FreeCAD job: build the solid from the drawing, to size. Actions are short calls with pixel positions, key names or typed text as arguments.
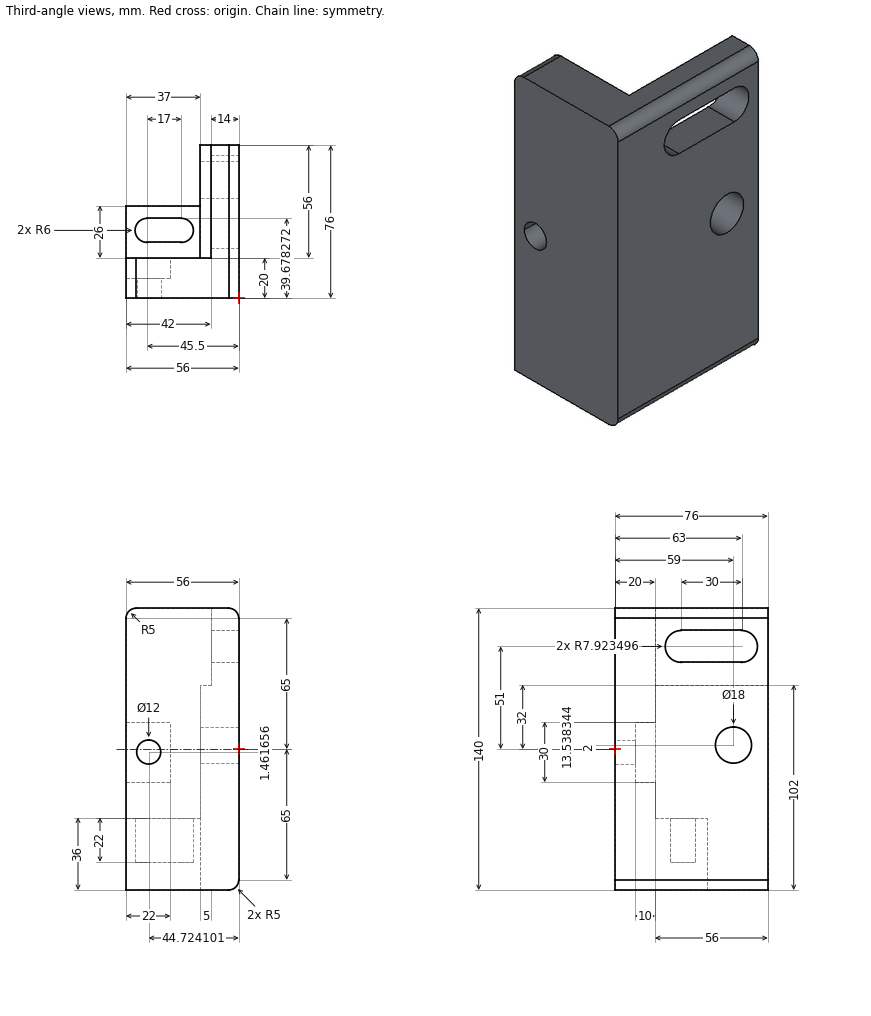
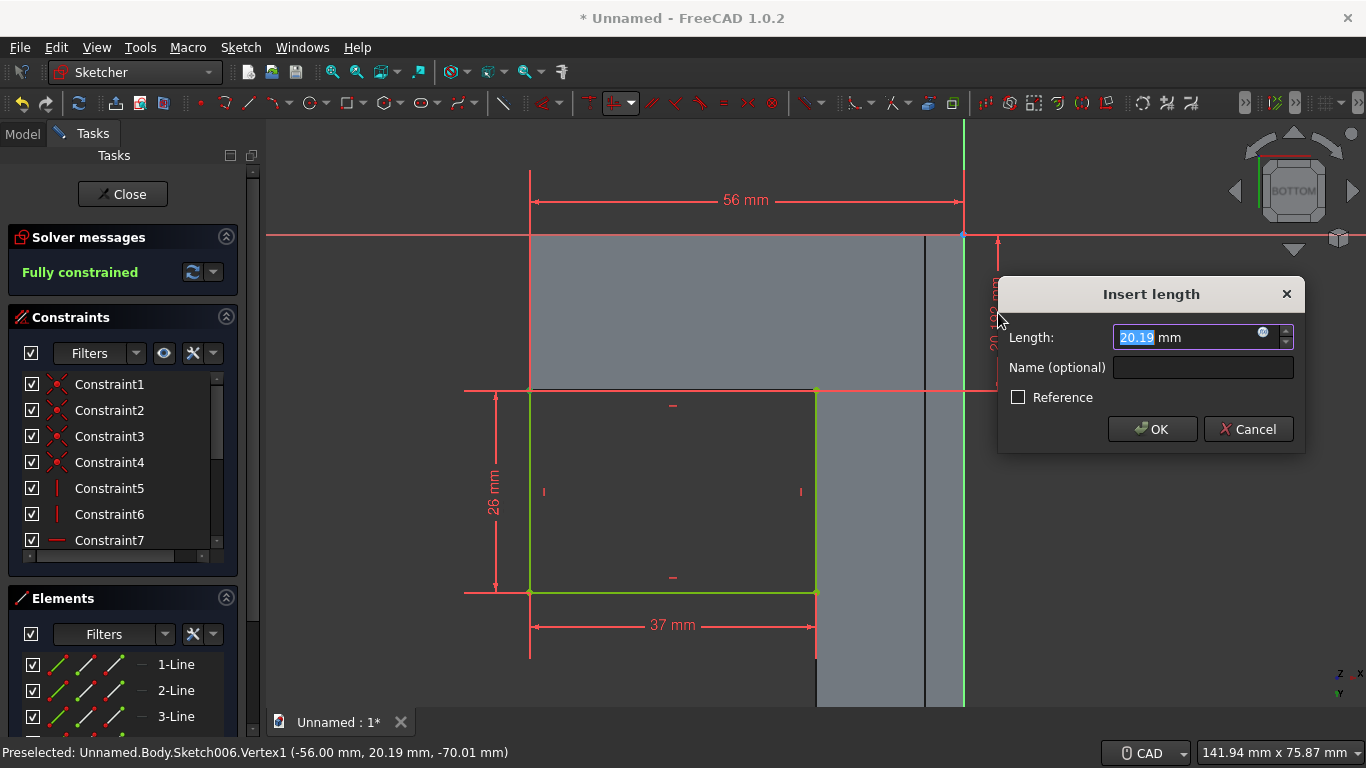
text(20)
key(Return)
key(Escape)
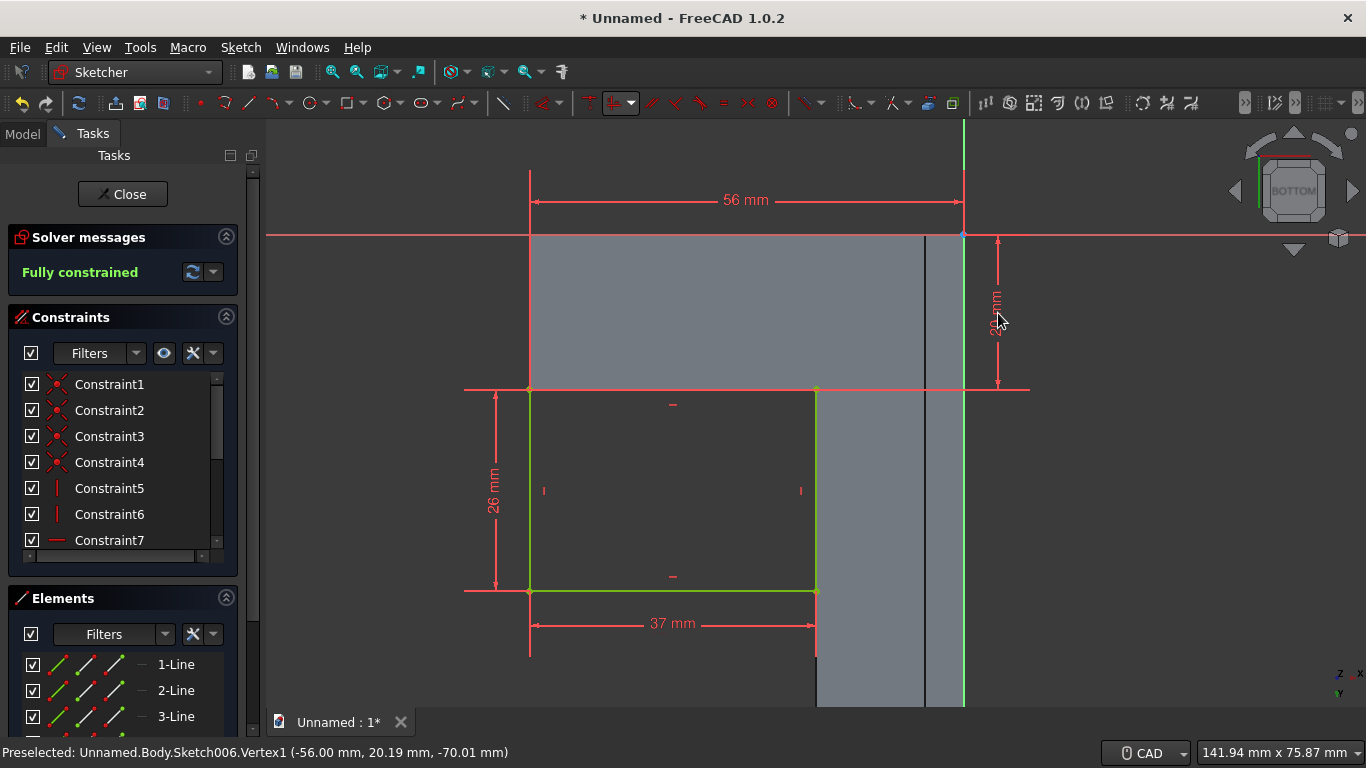
click(123, 194)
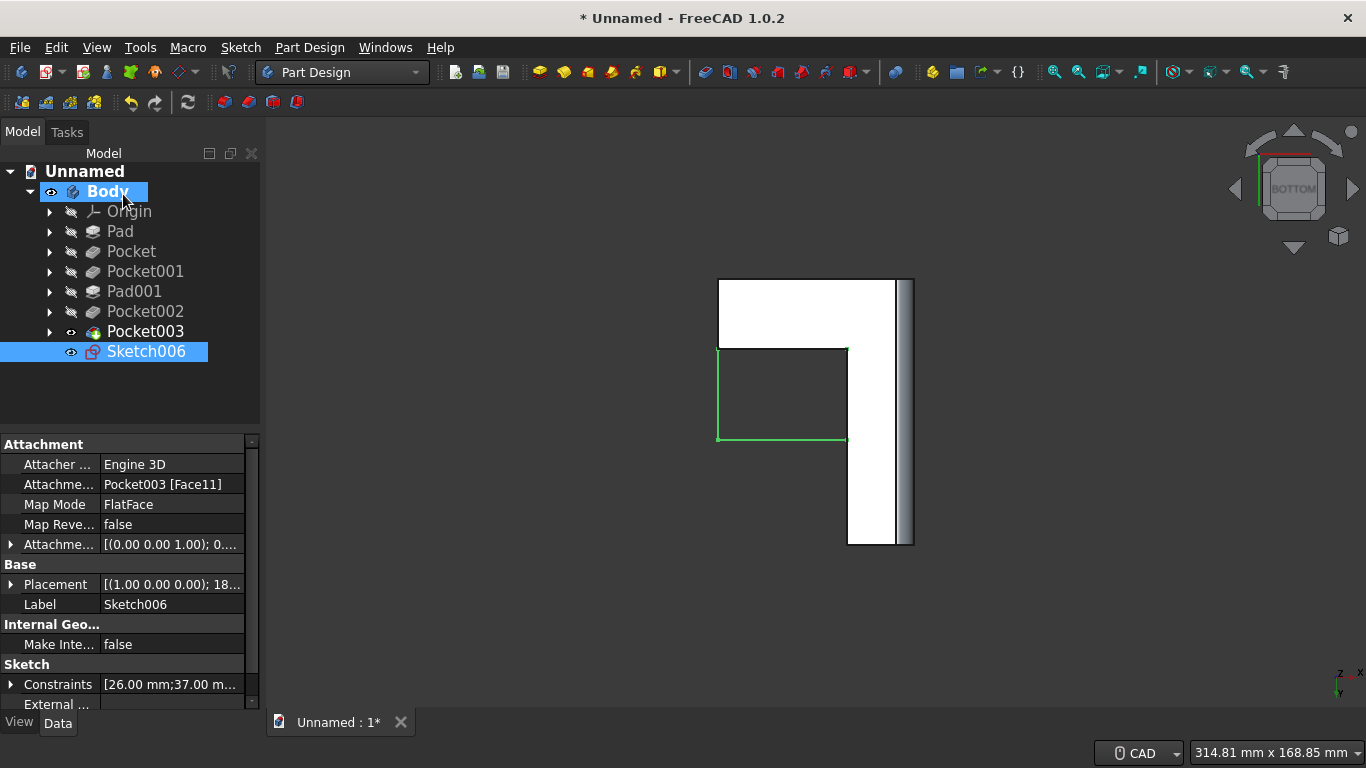
click(540, 72)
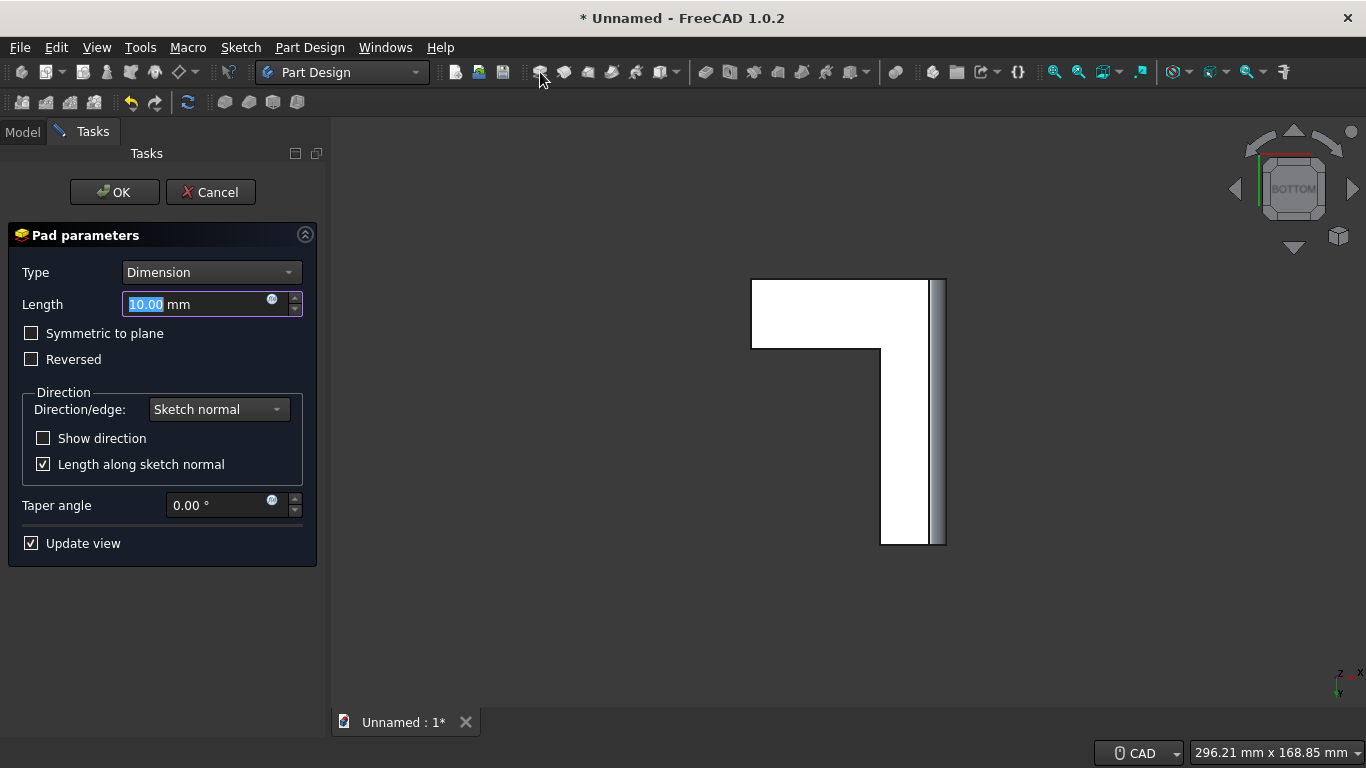
text(36)
key(Tab)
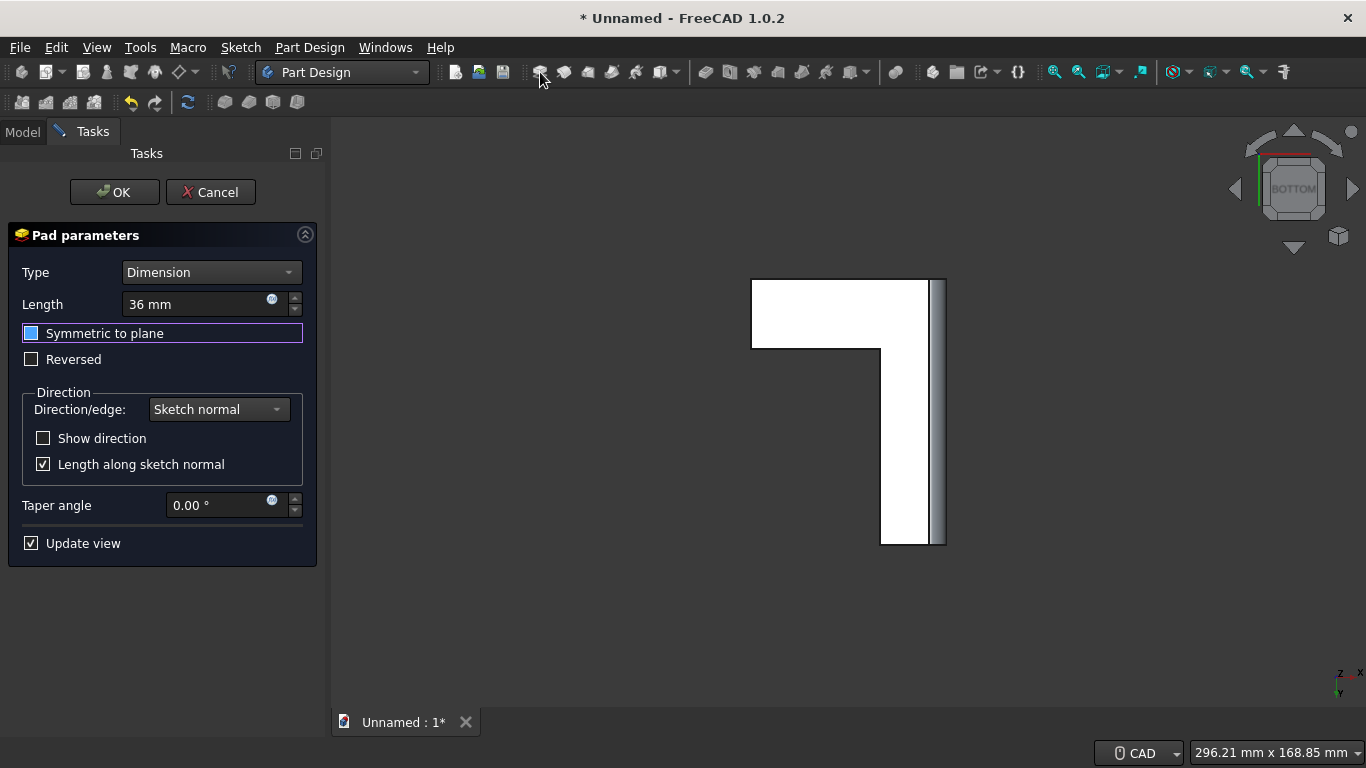
click(30, 359)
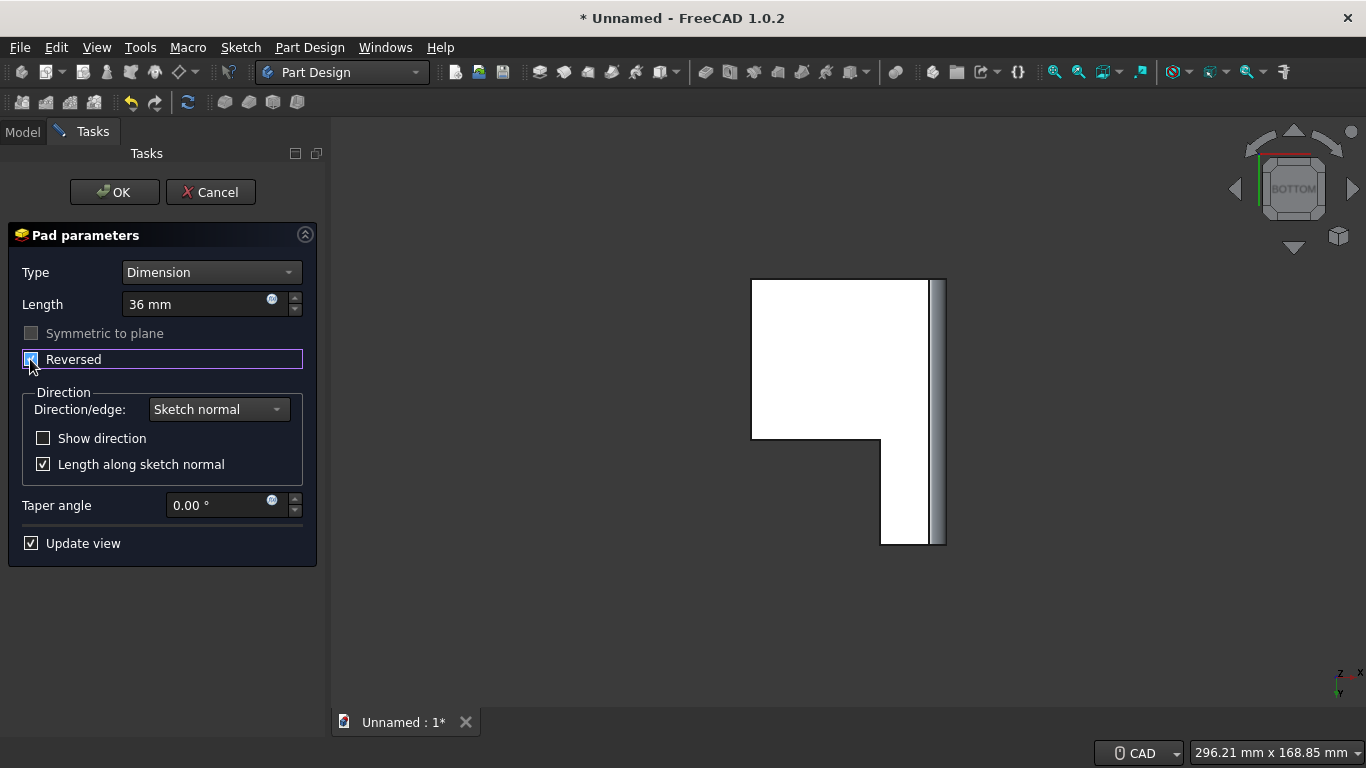
click(115, 192)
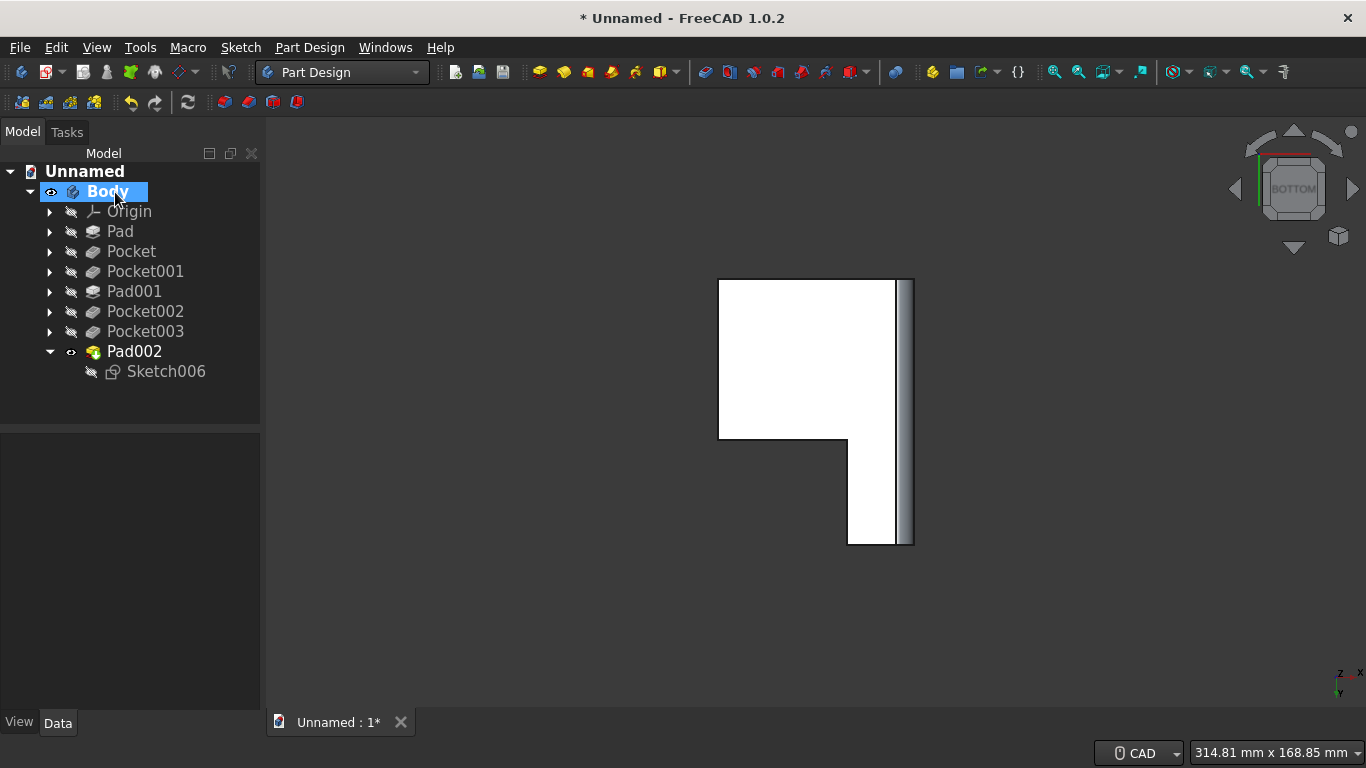
key(6)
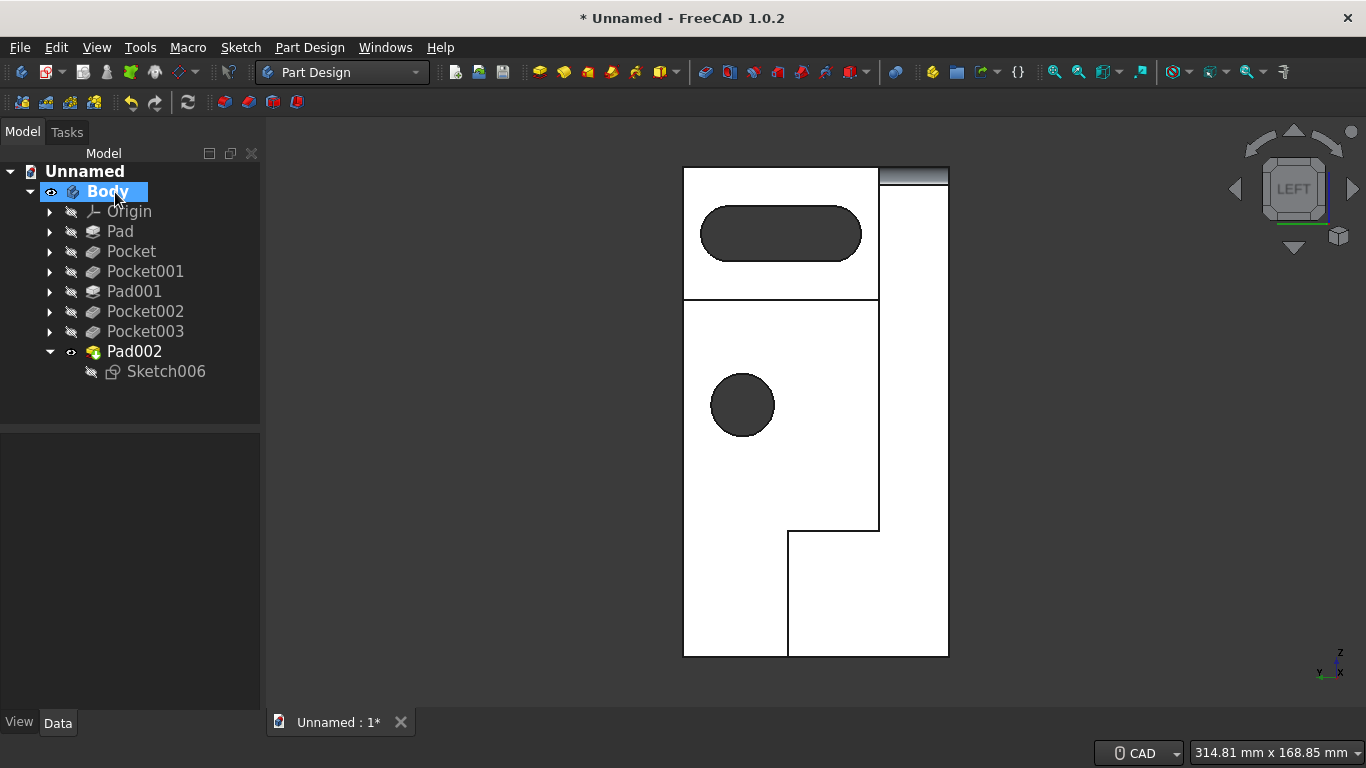
click(914, 285)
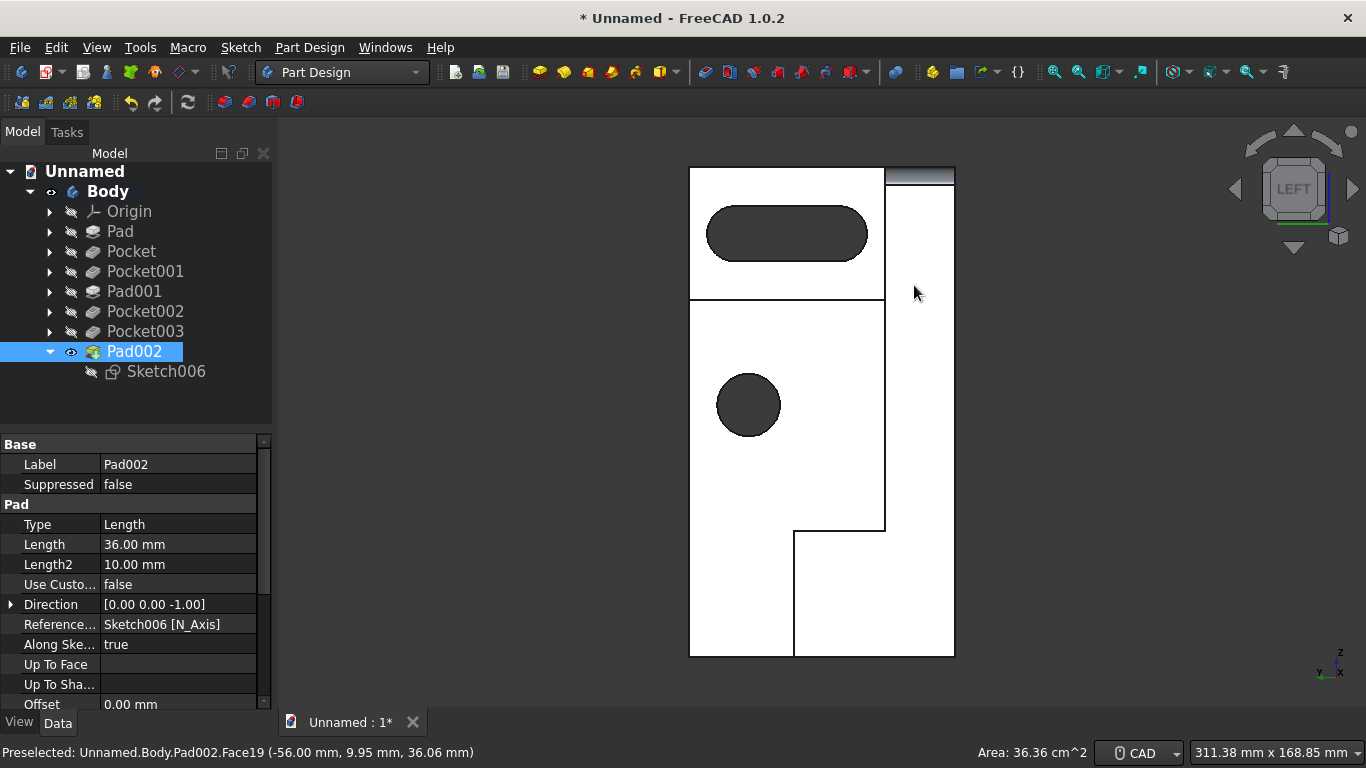
click(46, 72)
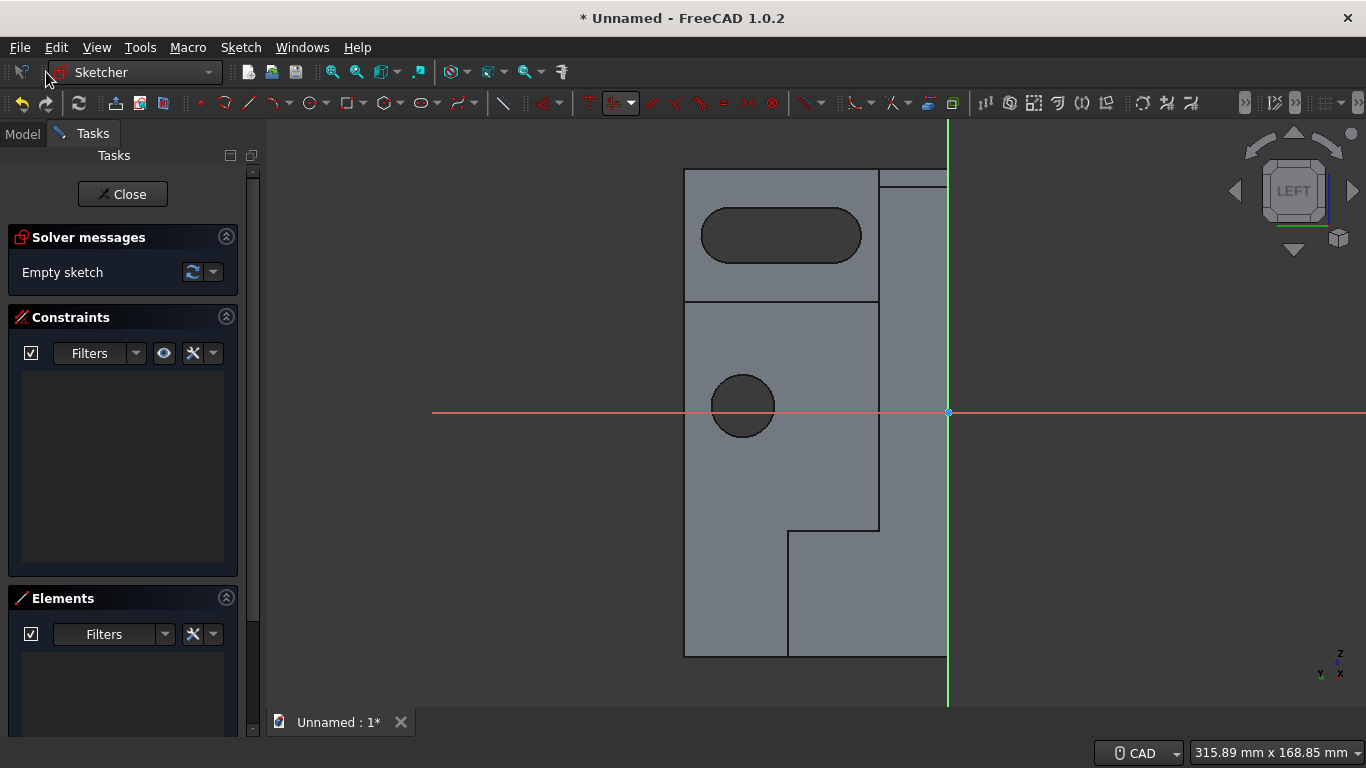
scroll(985, 420, up, 6)